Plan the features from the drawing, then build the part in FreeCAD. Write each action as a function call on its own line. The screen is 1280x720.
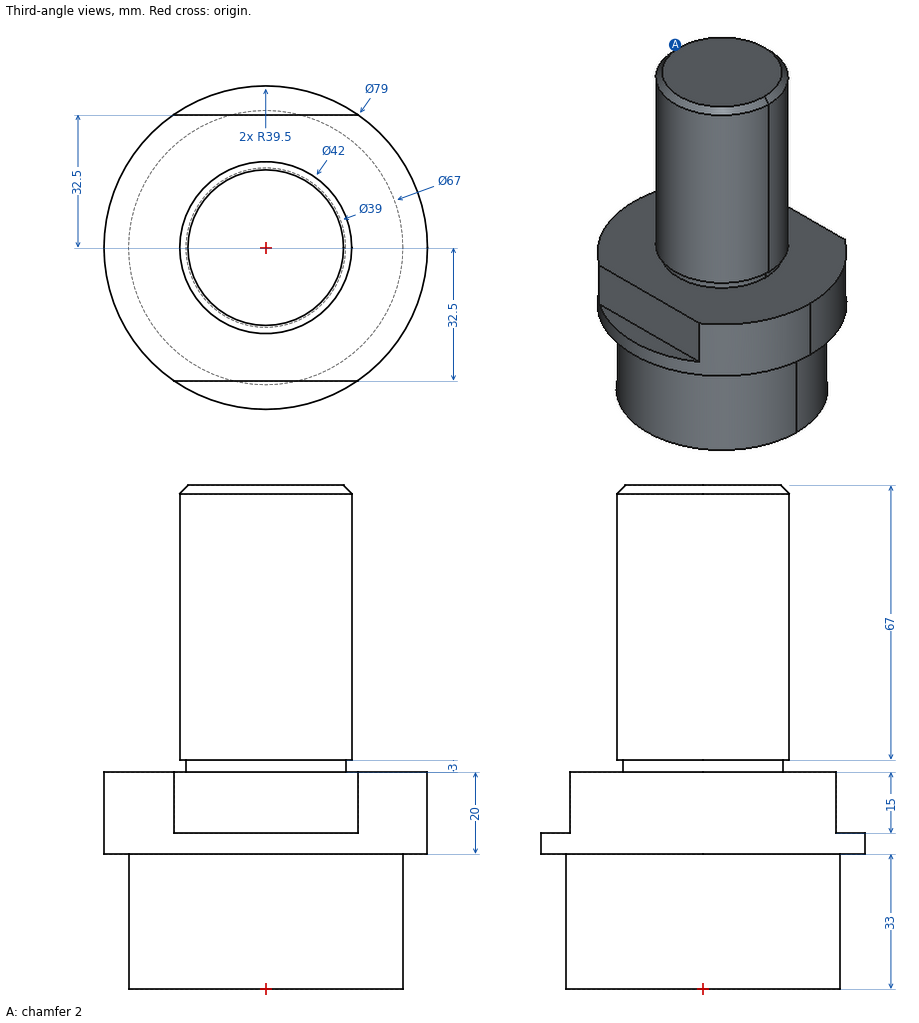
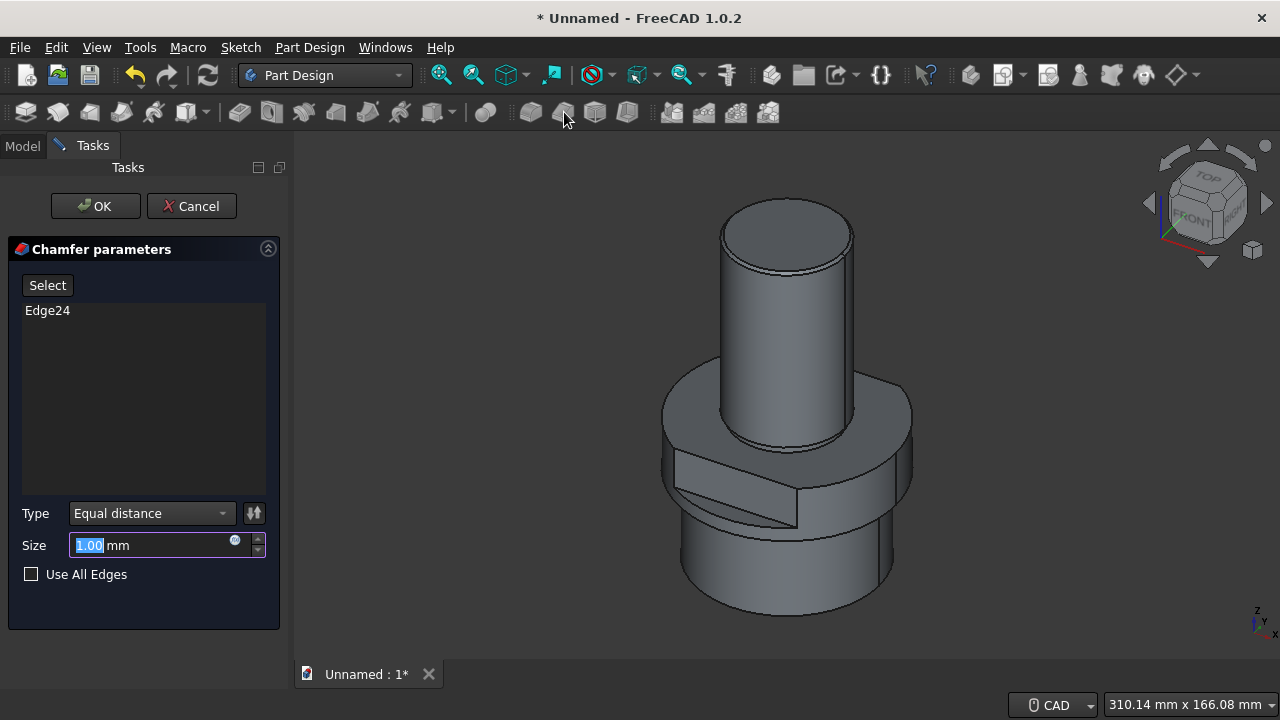
text(2)
key(Tab)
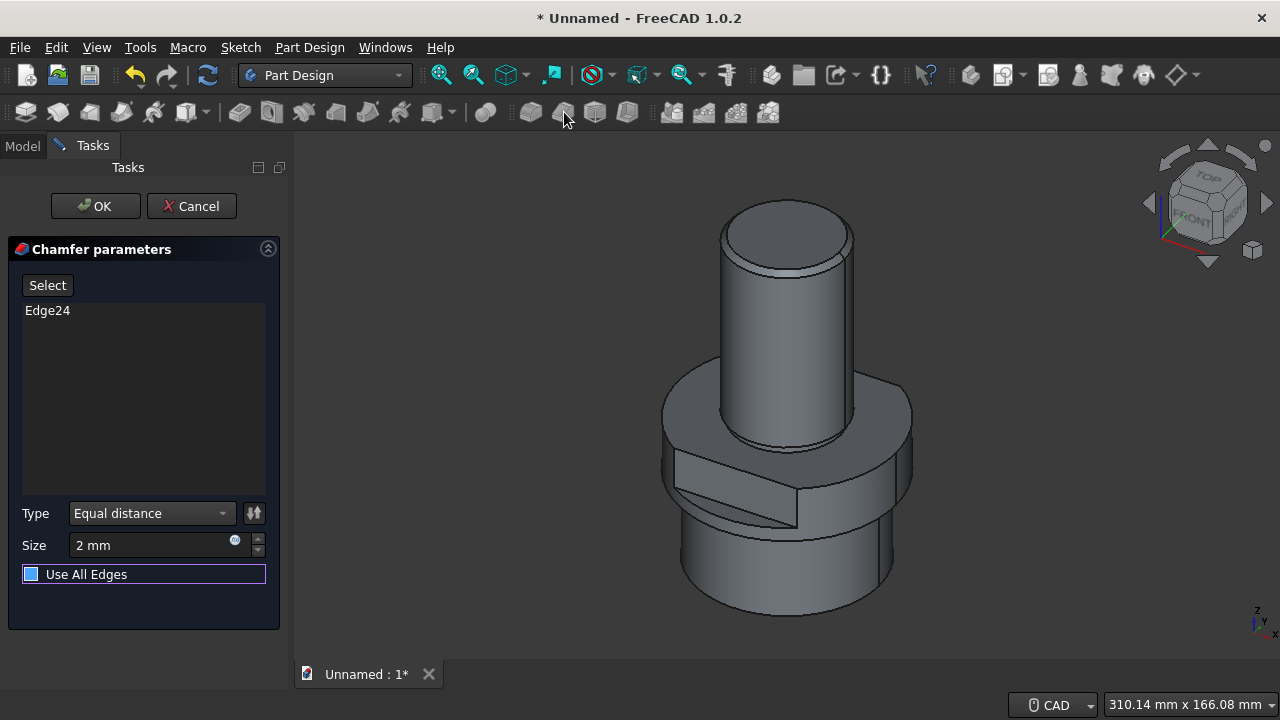
click(96, 206)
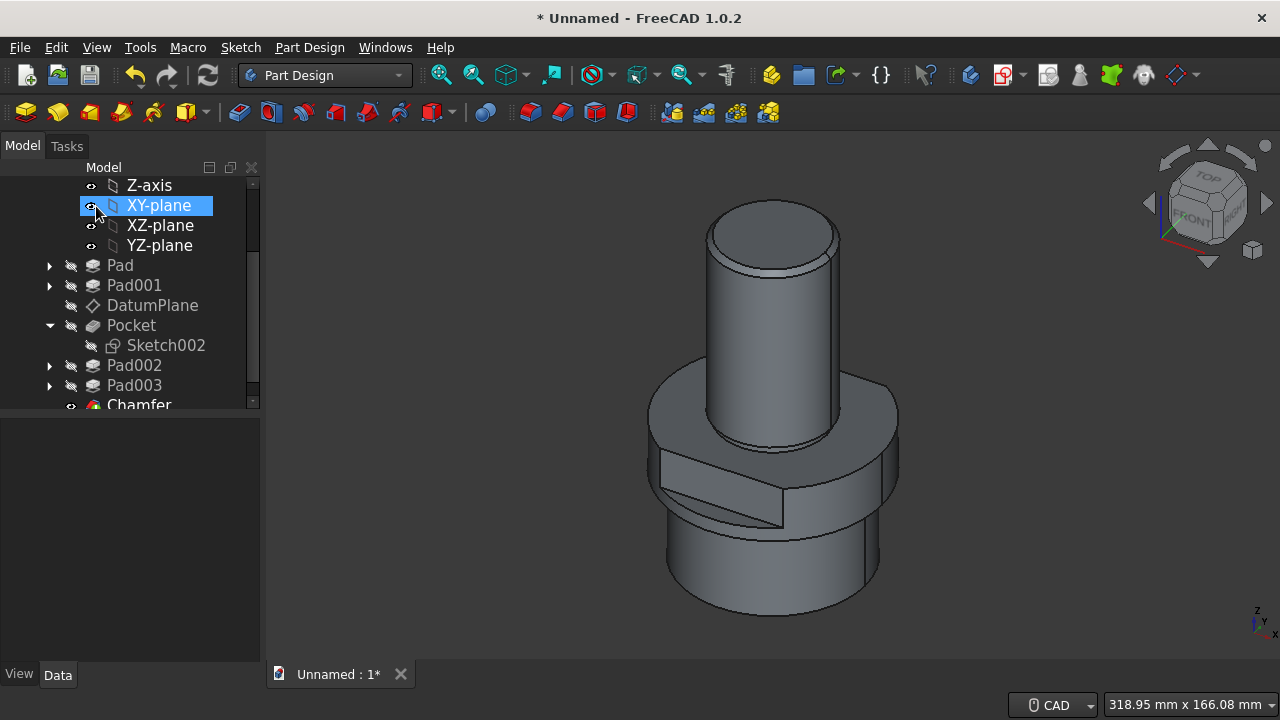
key(0)